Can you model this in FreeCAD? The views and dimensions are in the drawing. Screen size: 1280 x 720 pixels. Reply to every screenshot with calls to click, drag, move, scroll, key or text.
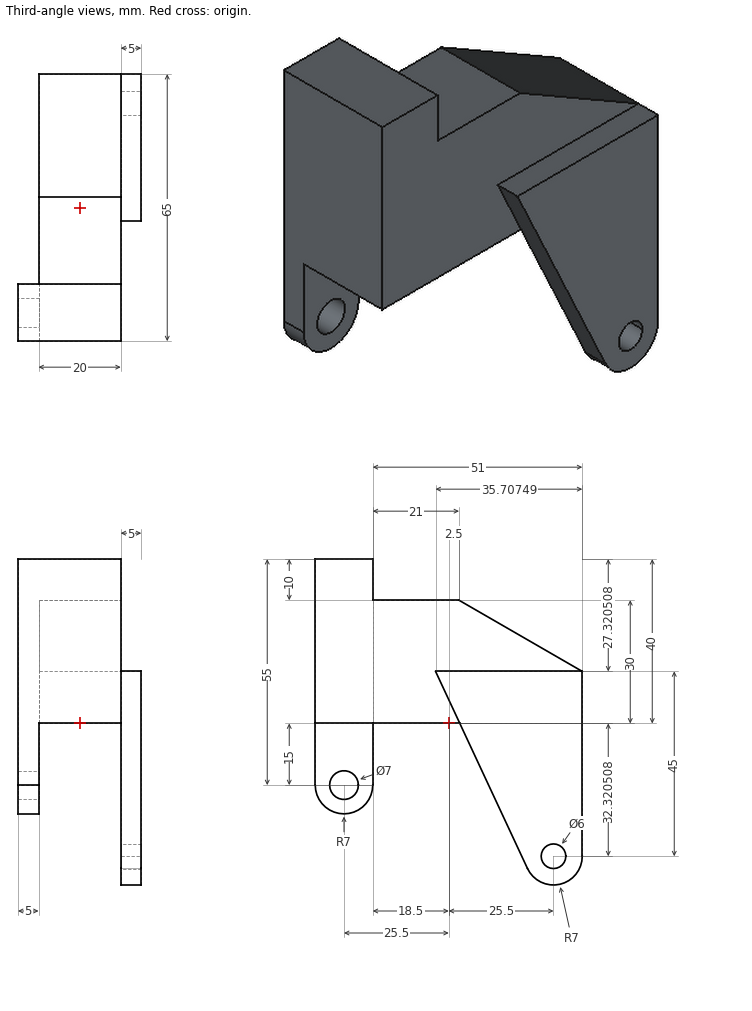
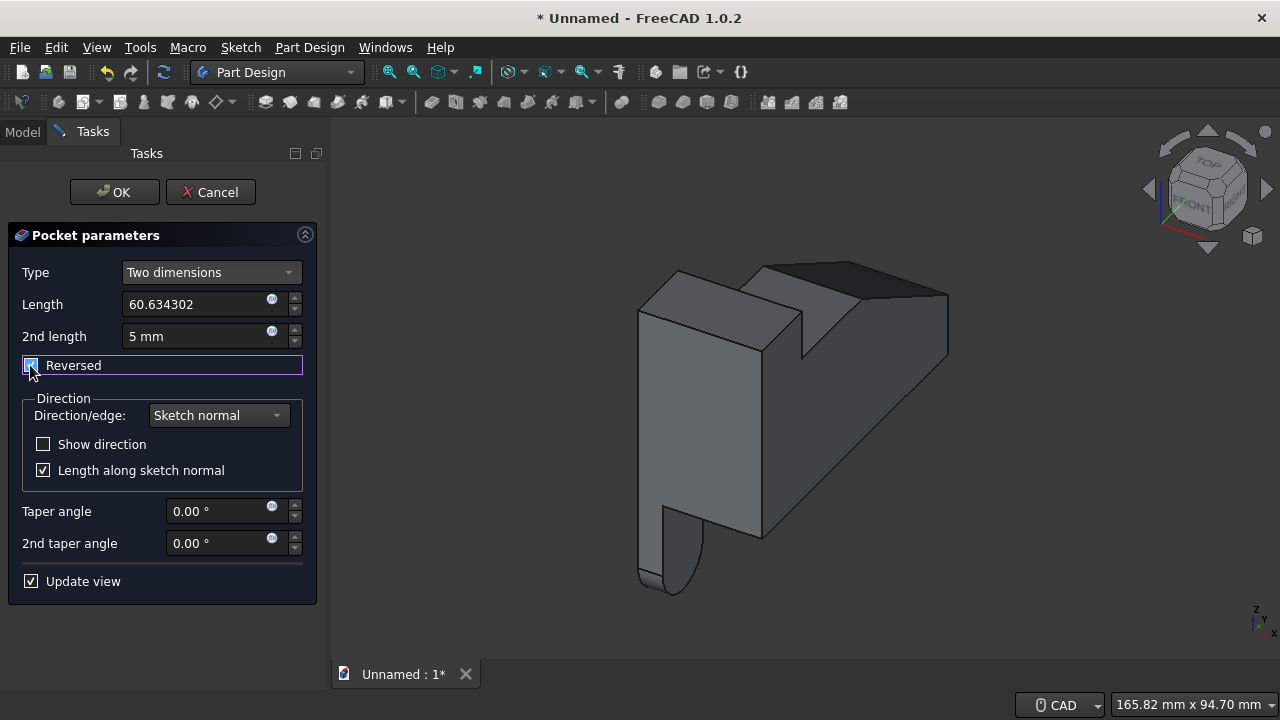
click(115, 192)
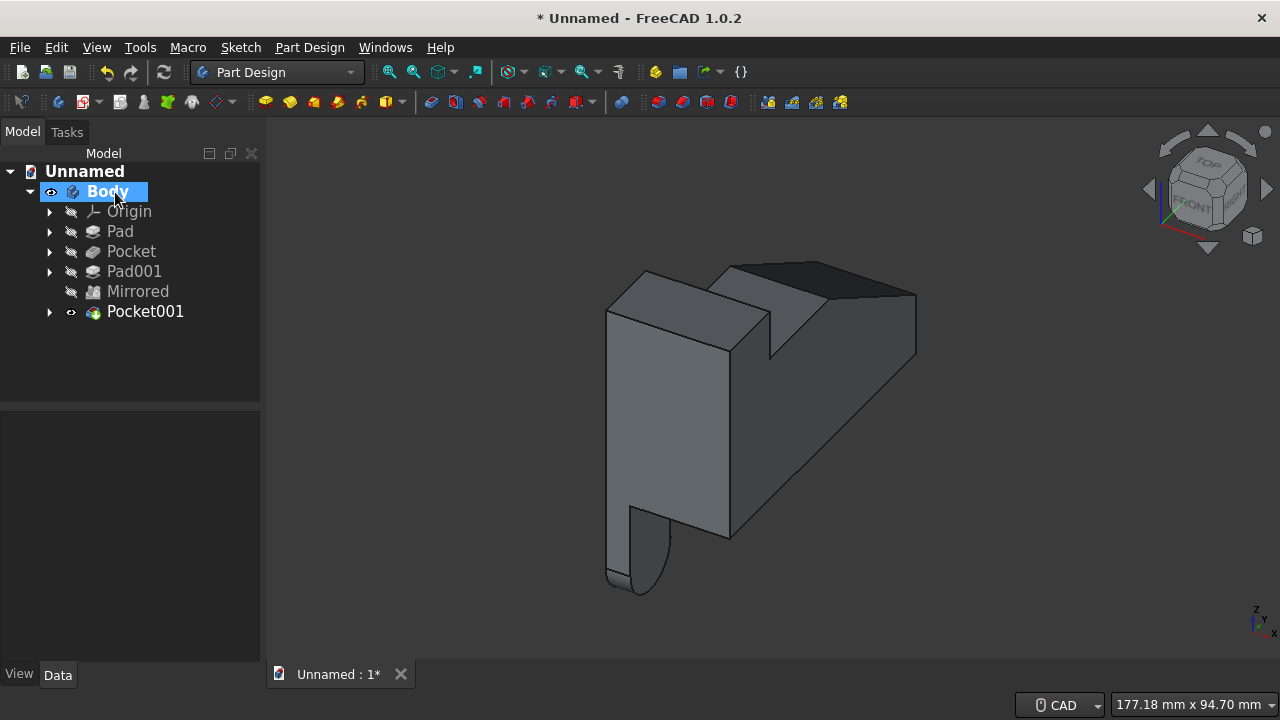
key(6)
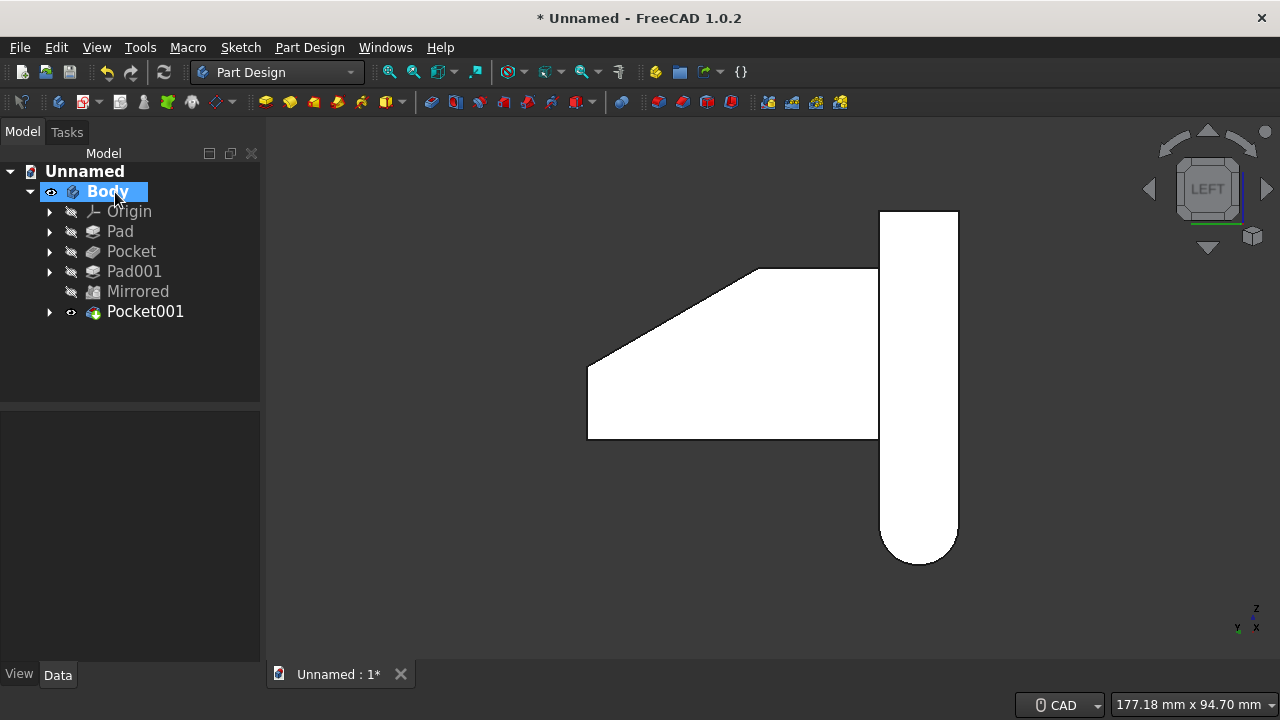
click(775, 353)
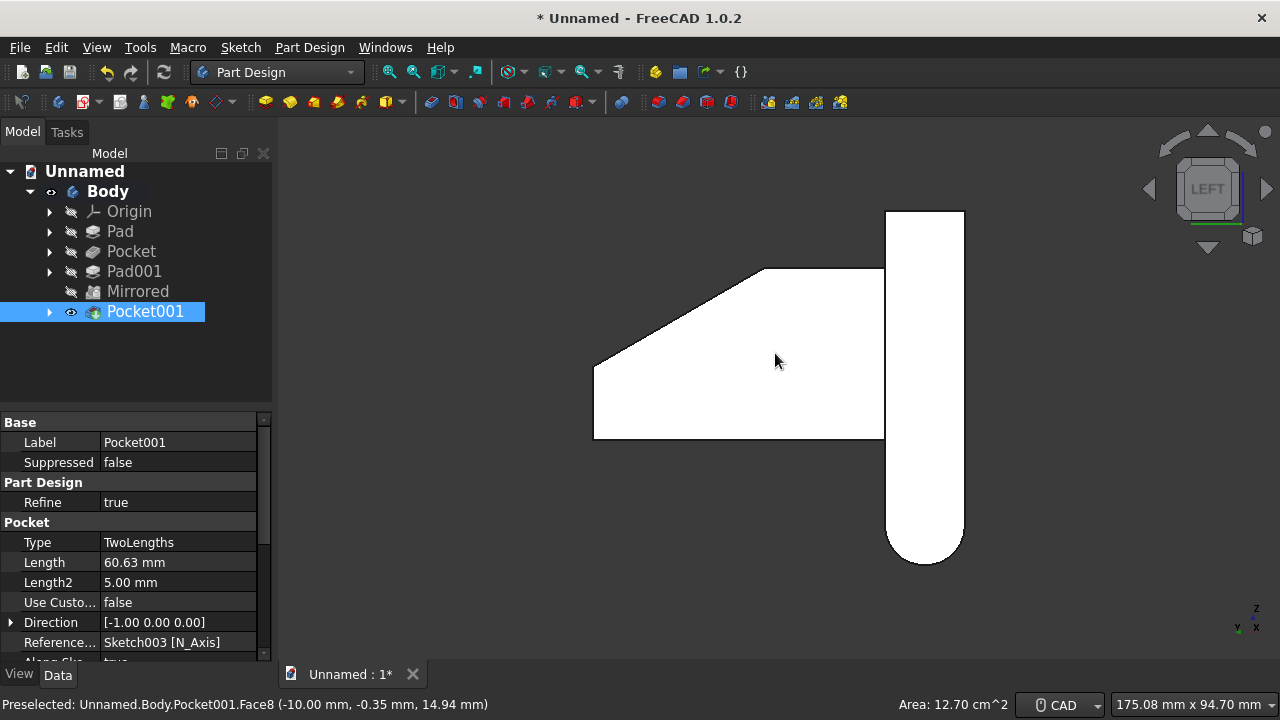
click(84, 102)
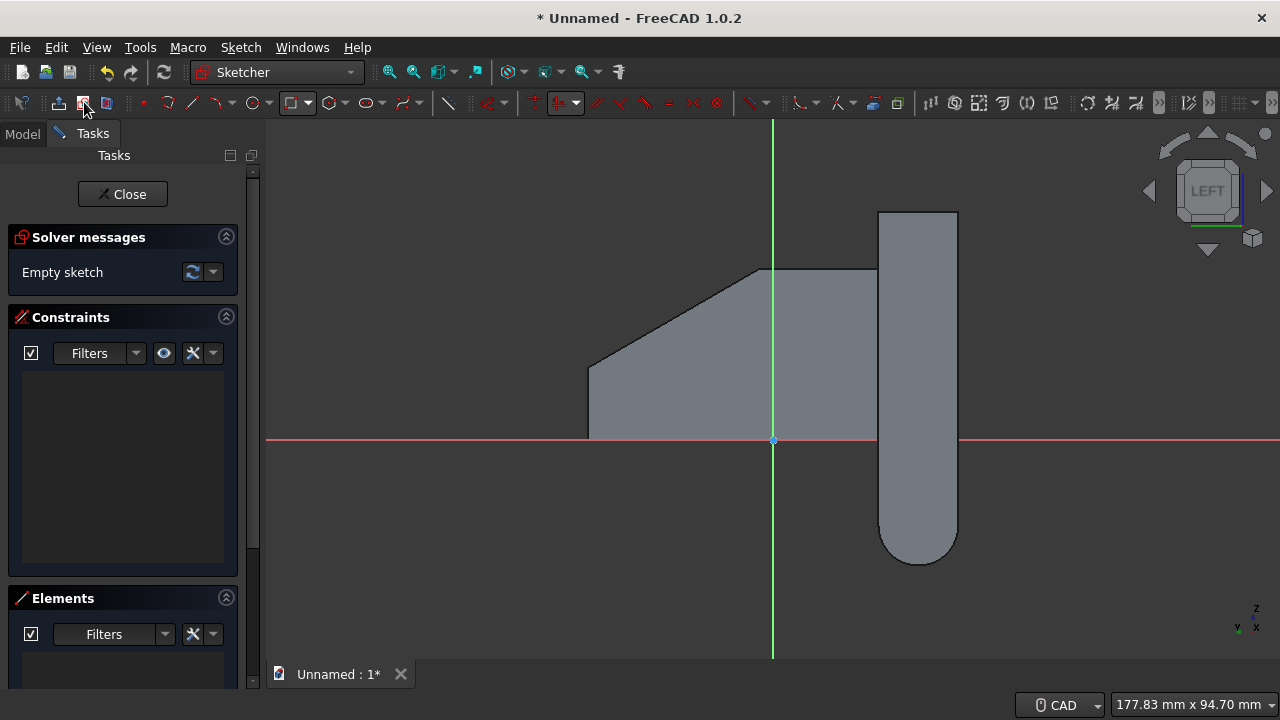
key(q)
key(s)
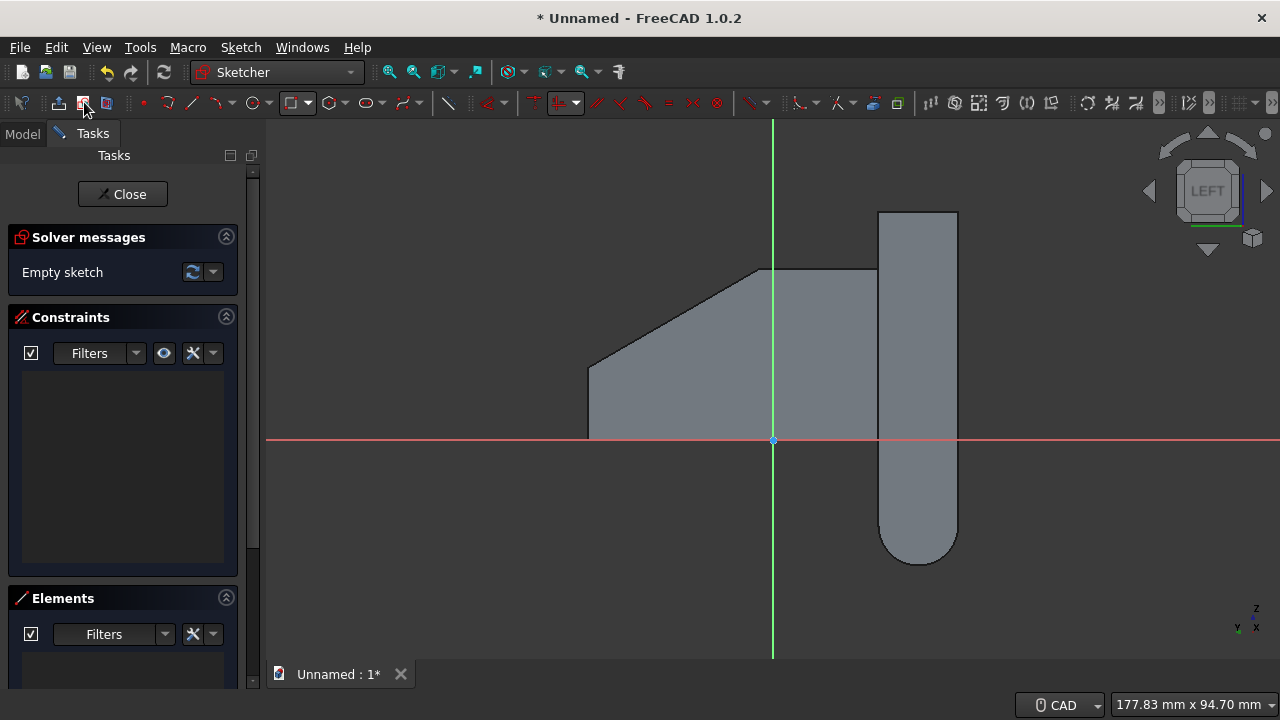
scroll(945, 543, up, 11)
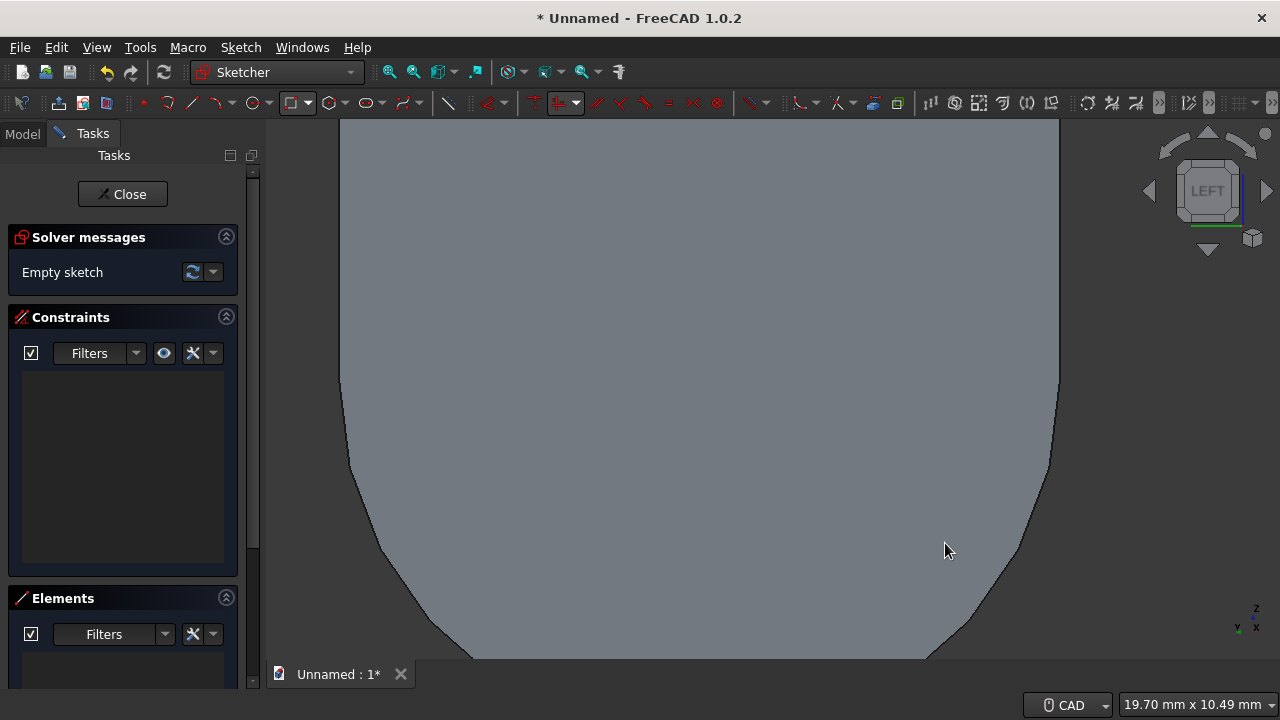
key(g)
key(c)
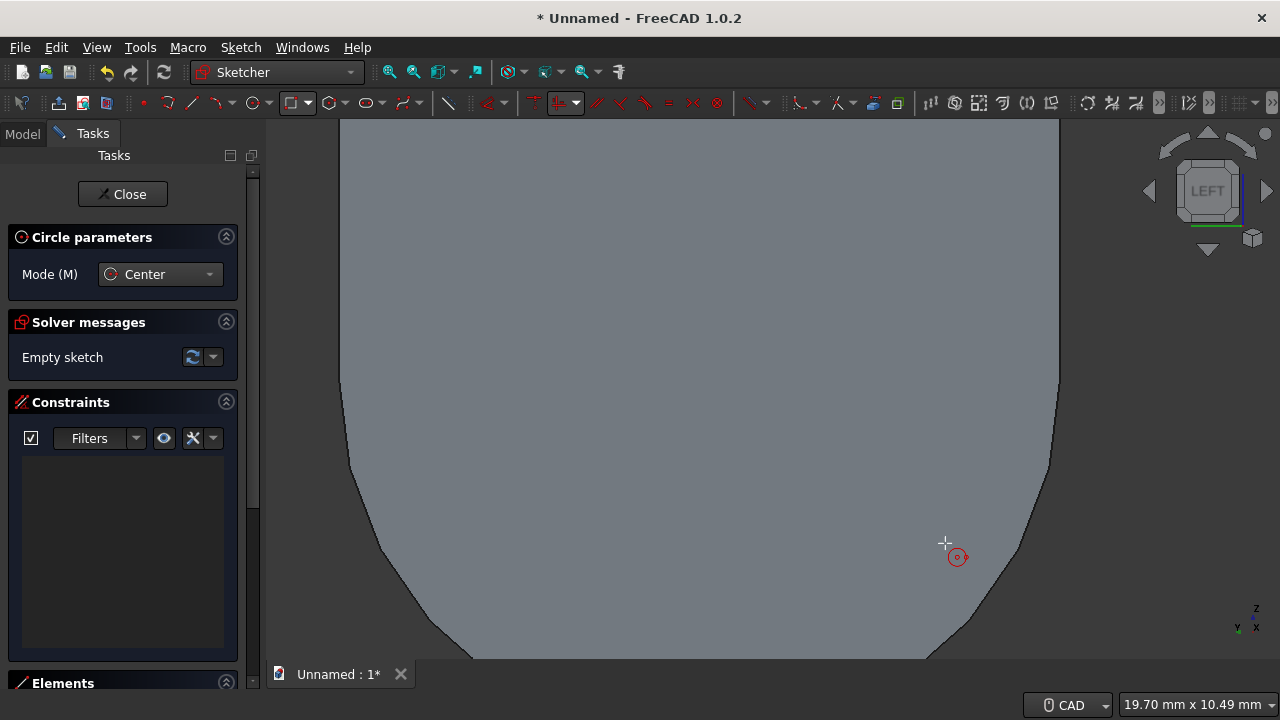
click(700, 382)
move(827, 255)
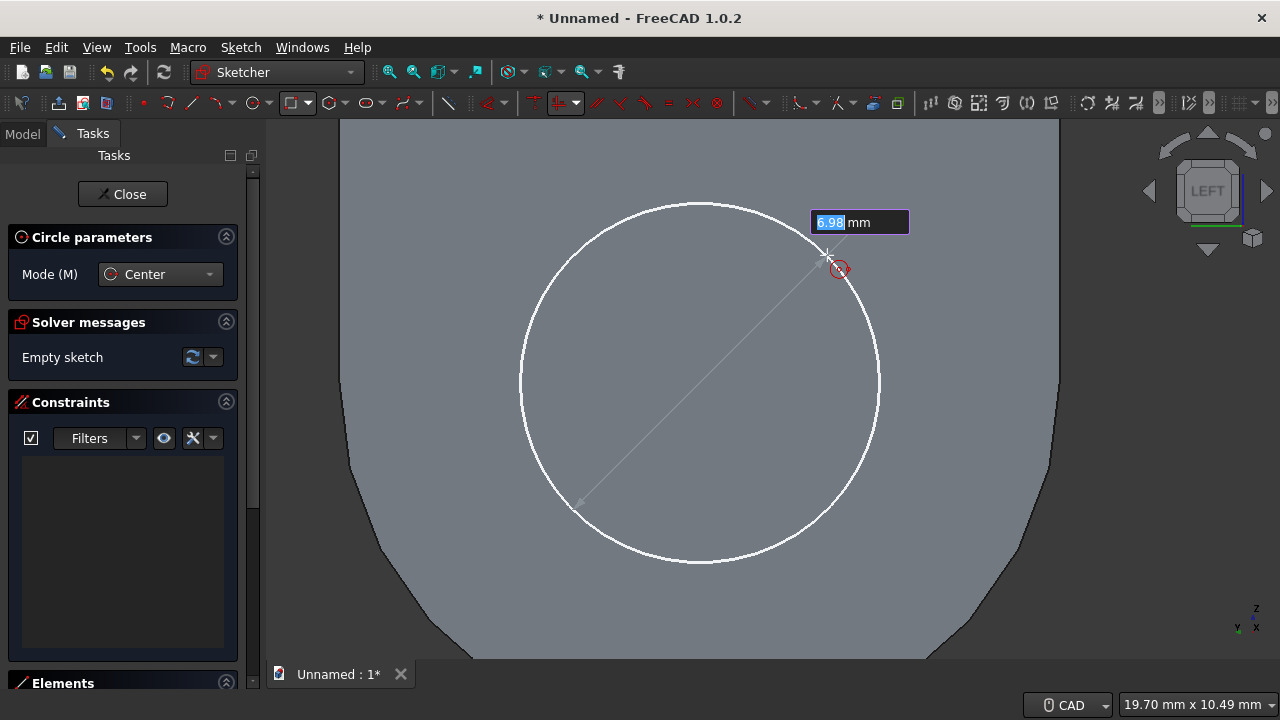
text(7)
key(Return)
key(Escape)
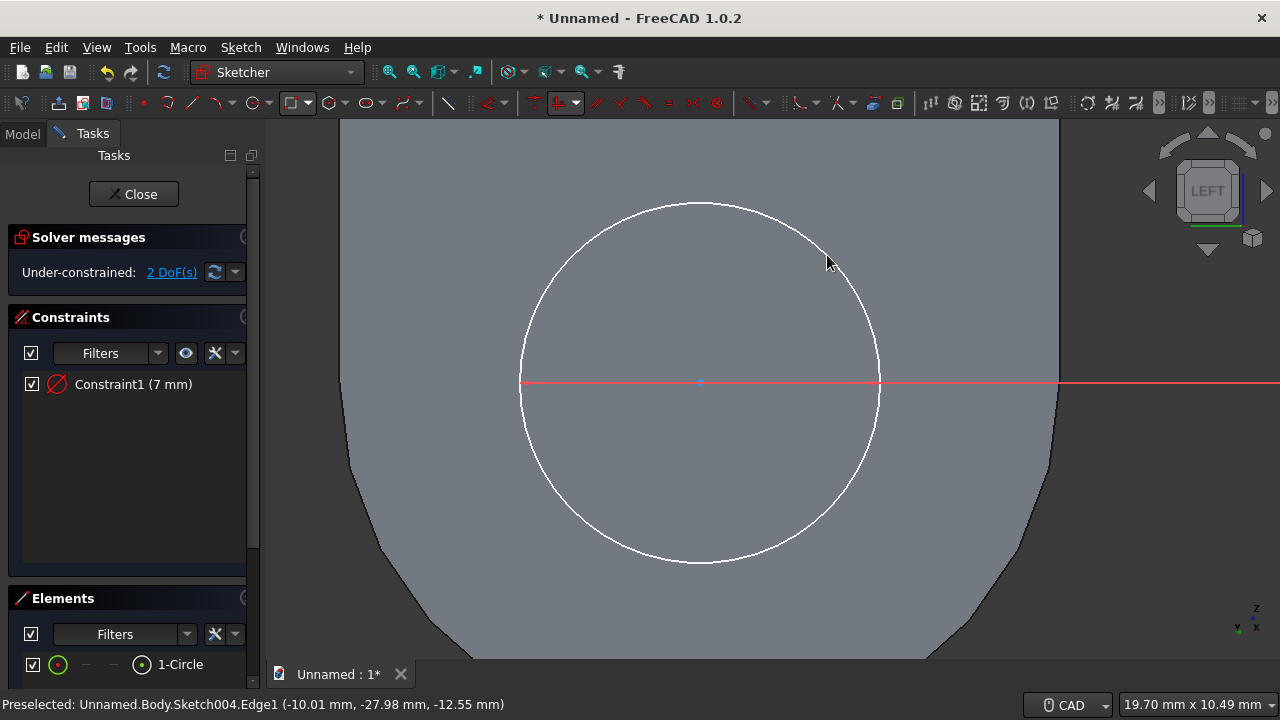
key(d)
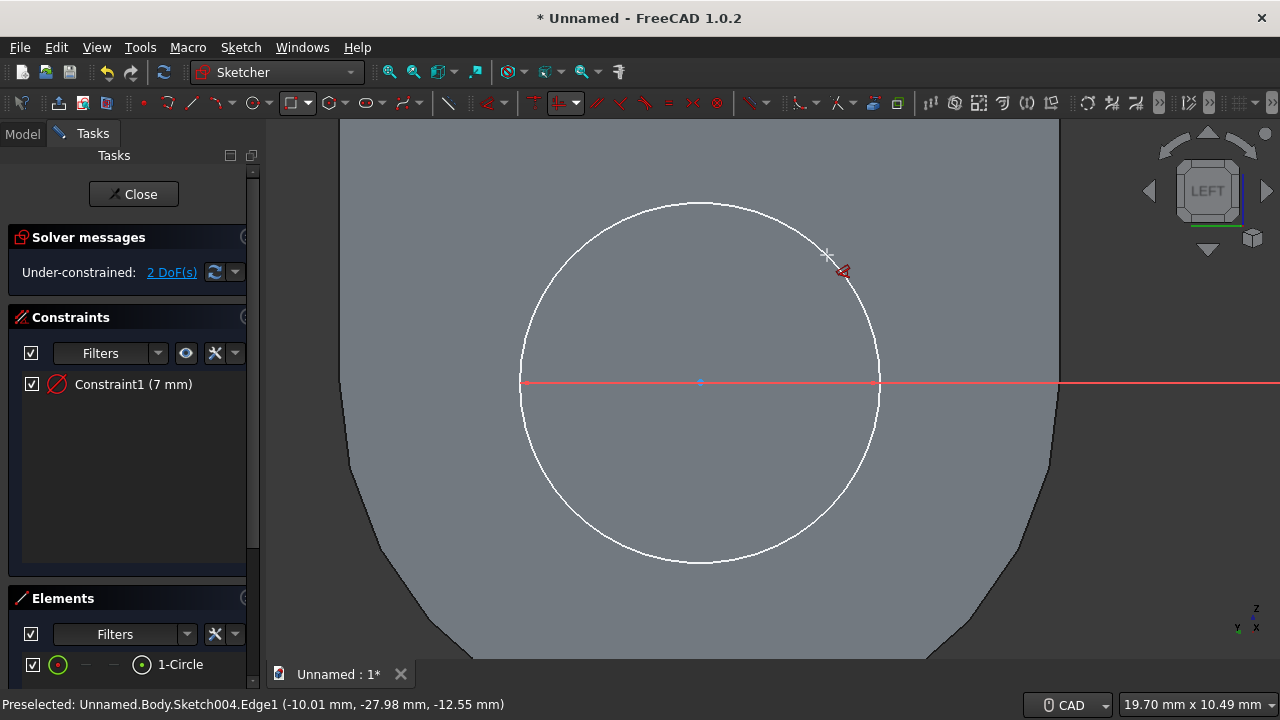
click(700, 383)
click(734, 265)